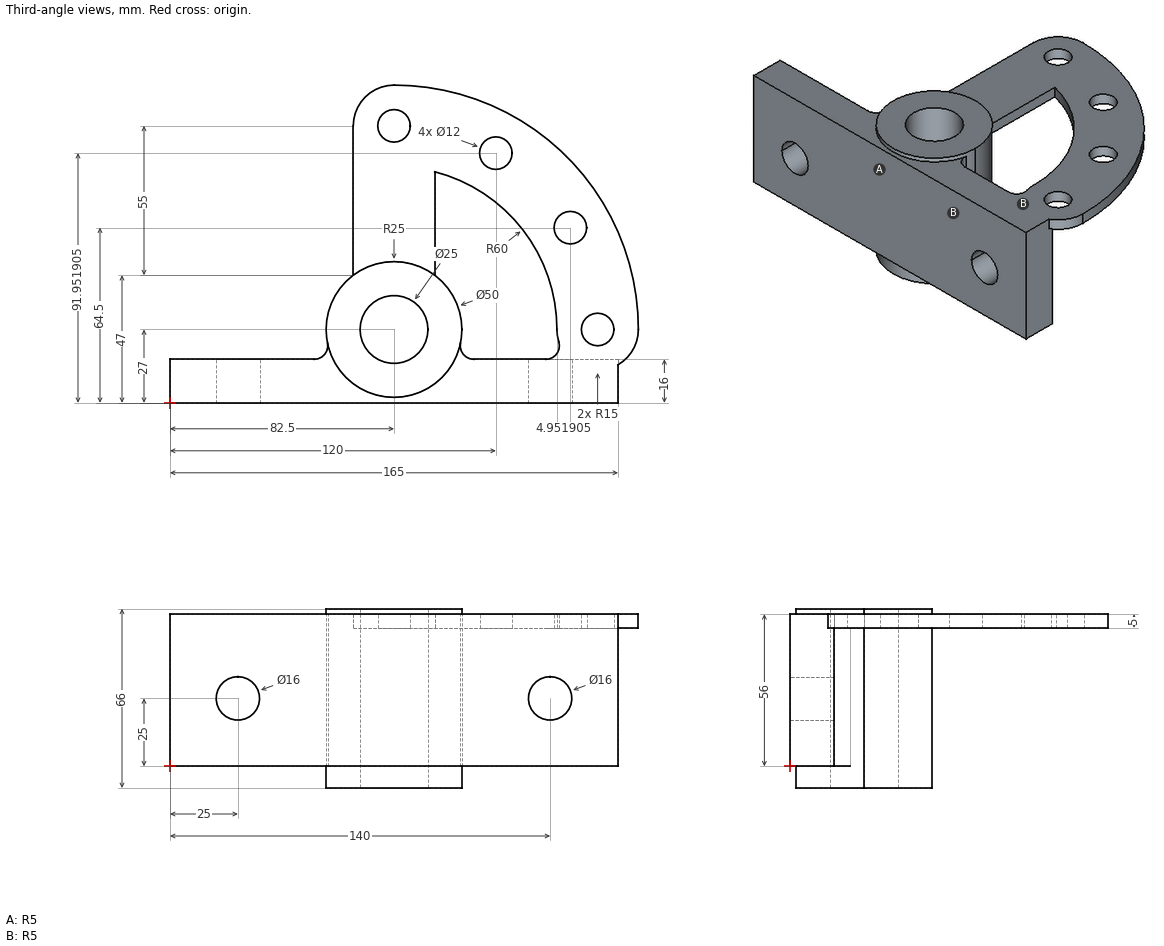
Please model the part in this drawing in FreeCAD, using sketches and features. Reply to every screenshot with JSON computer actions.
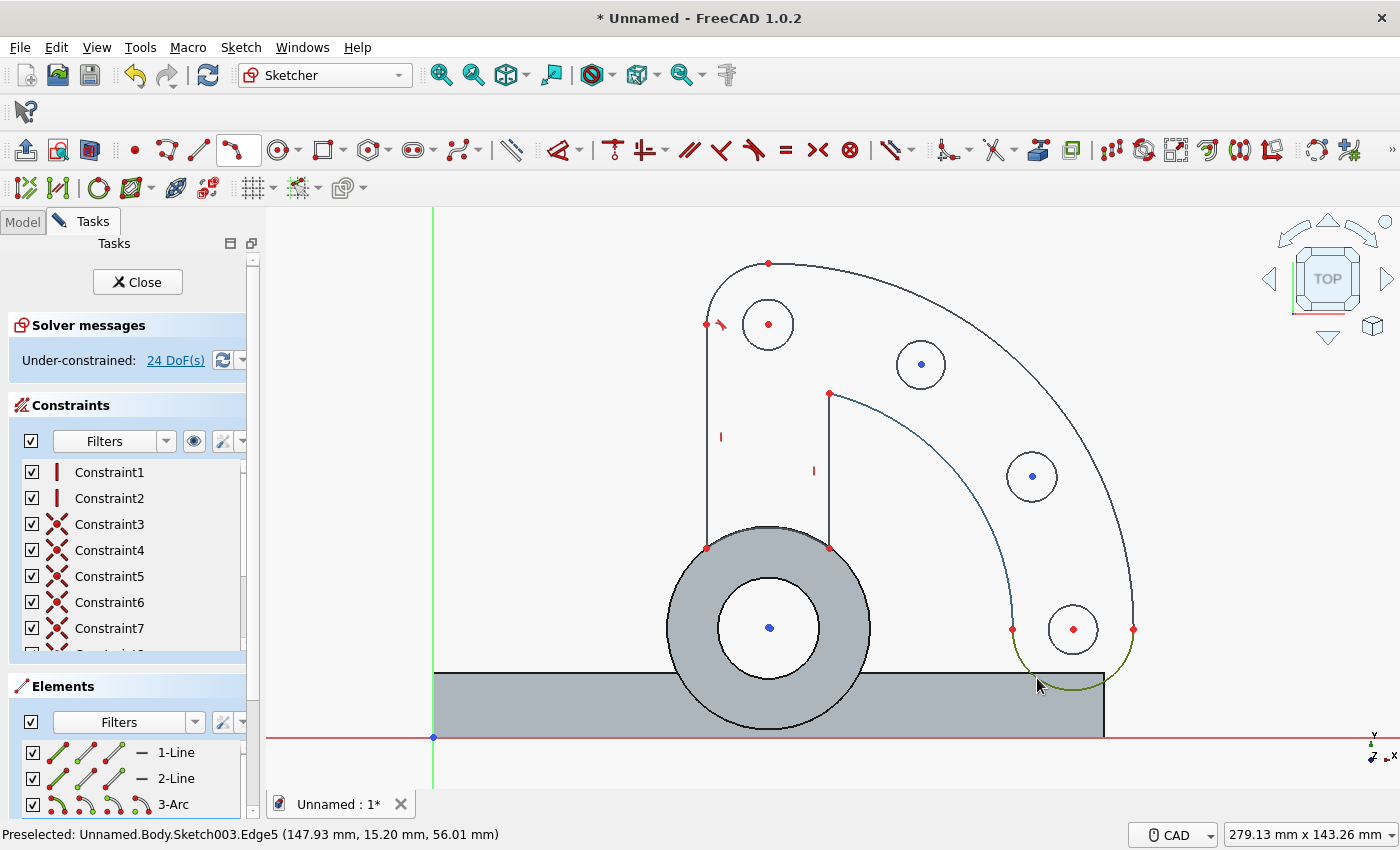
{"action": "left_click", "coordinate": [754, 150]}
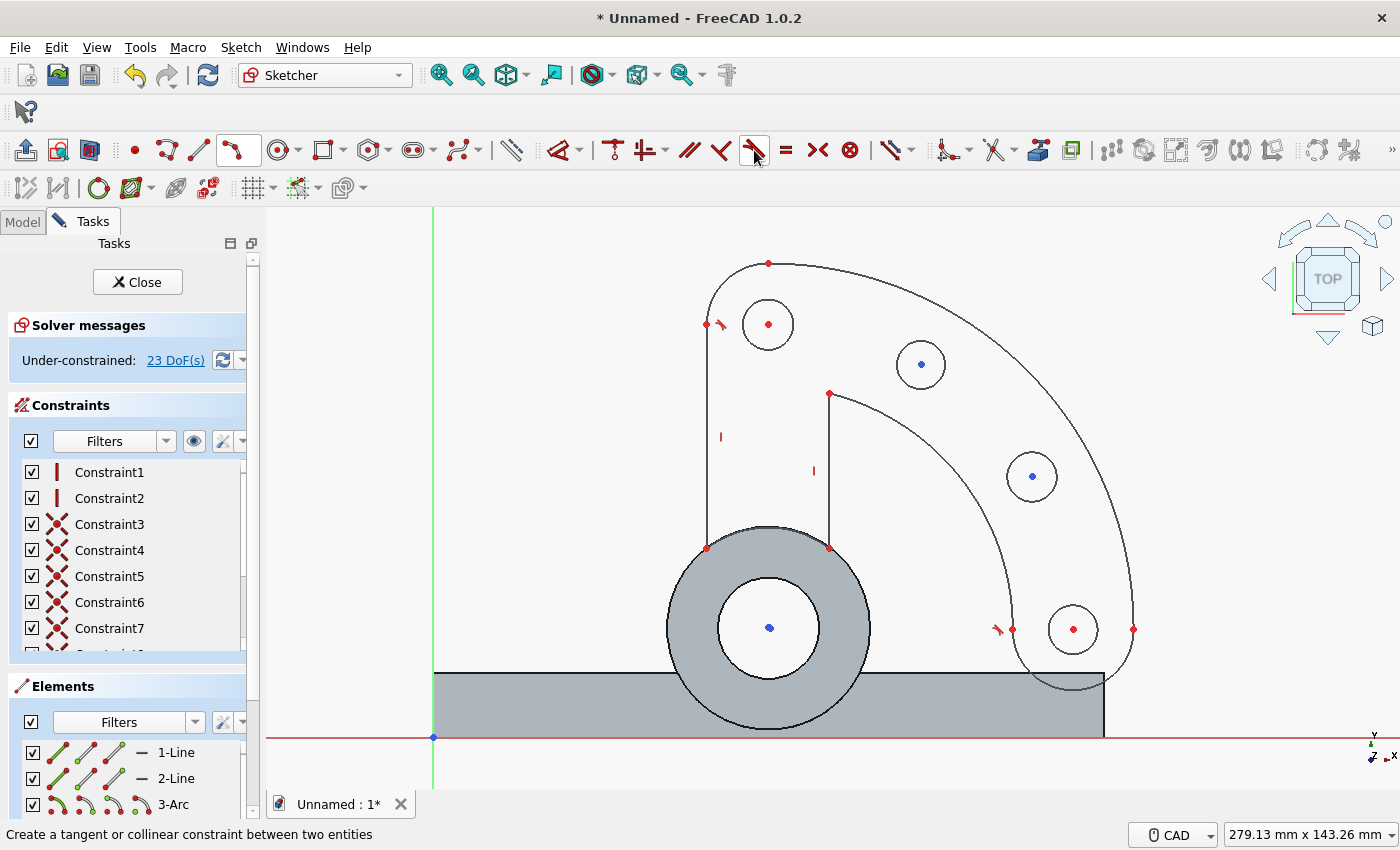
{"action": "left_click", "coordinate": [1038, 679]}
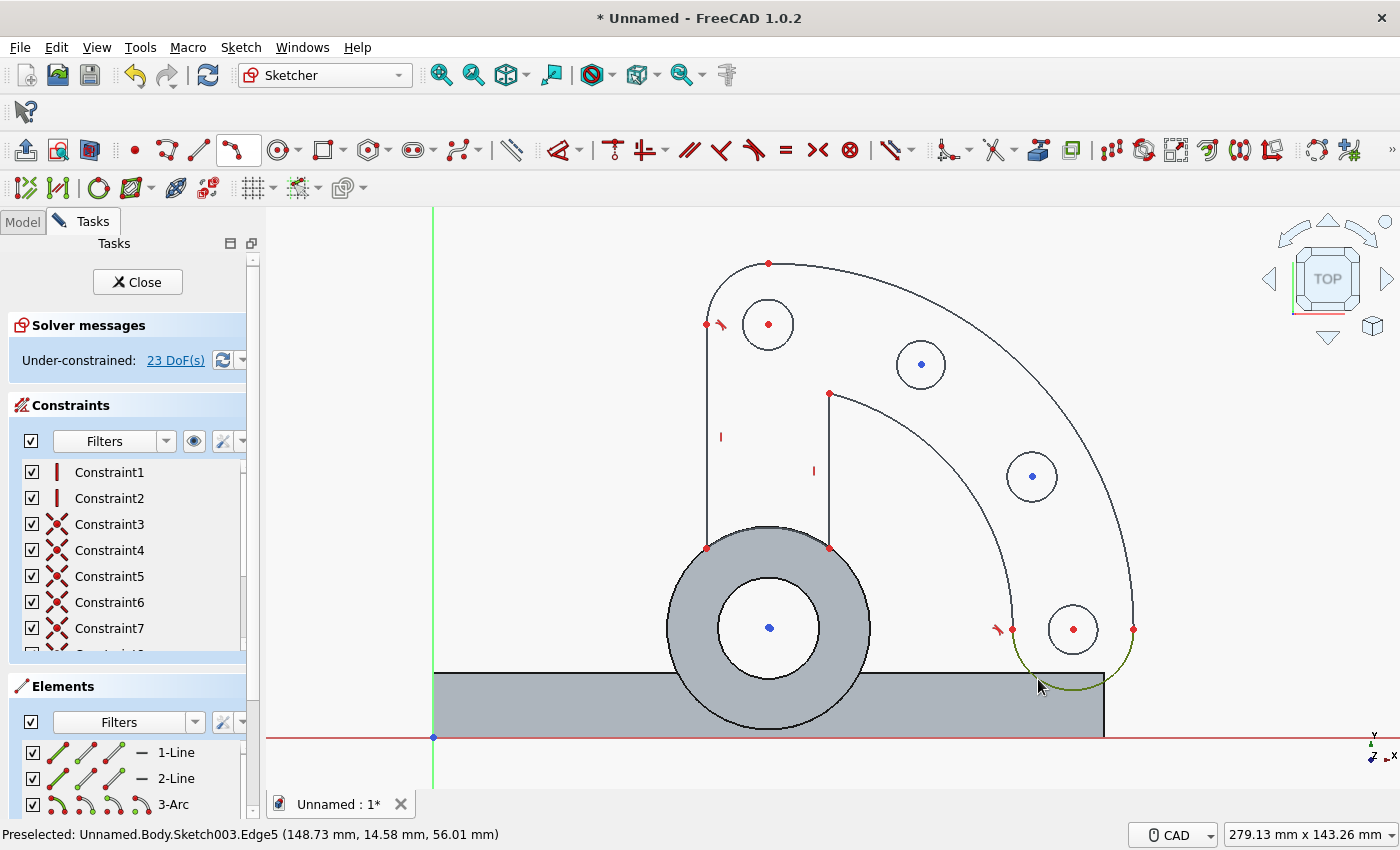
{"action": "left_click", "coordinate": [1094, 463]}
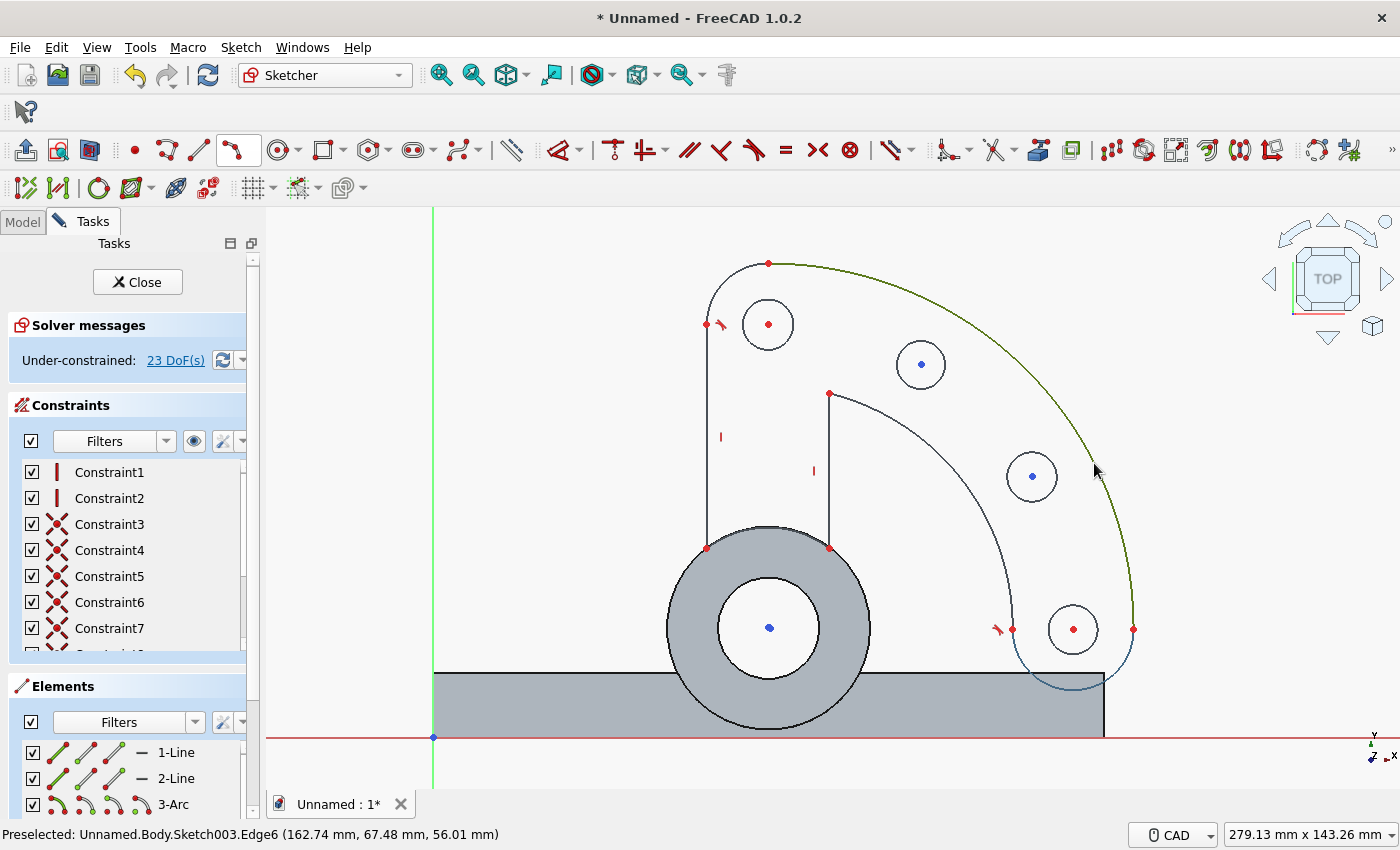
{"action": "left_click", "coordinate": [754, 150]}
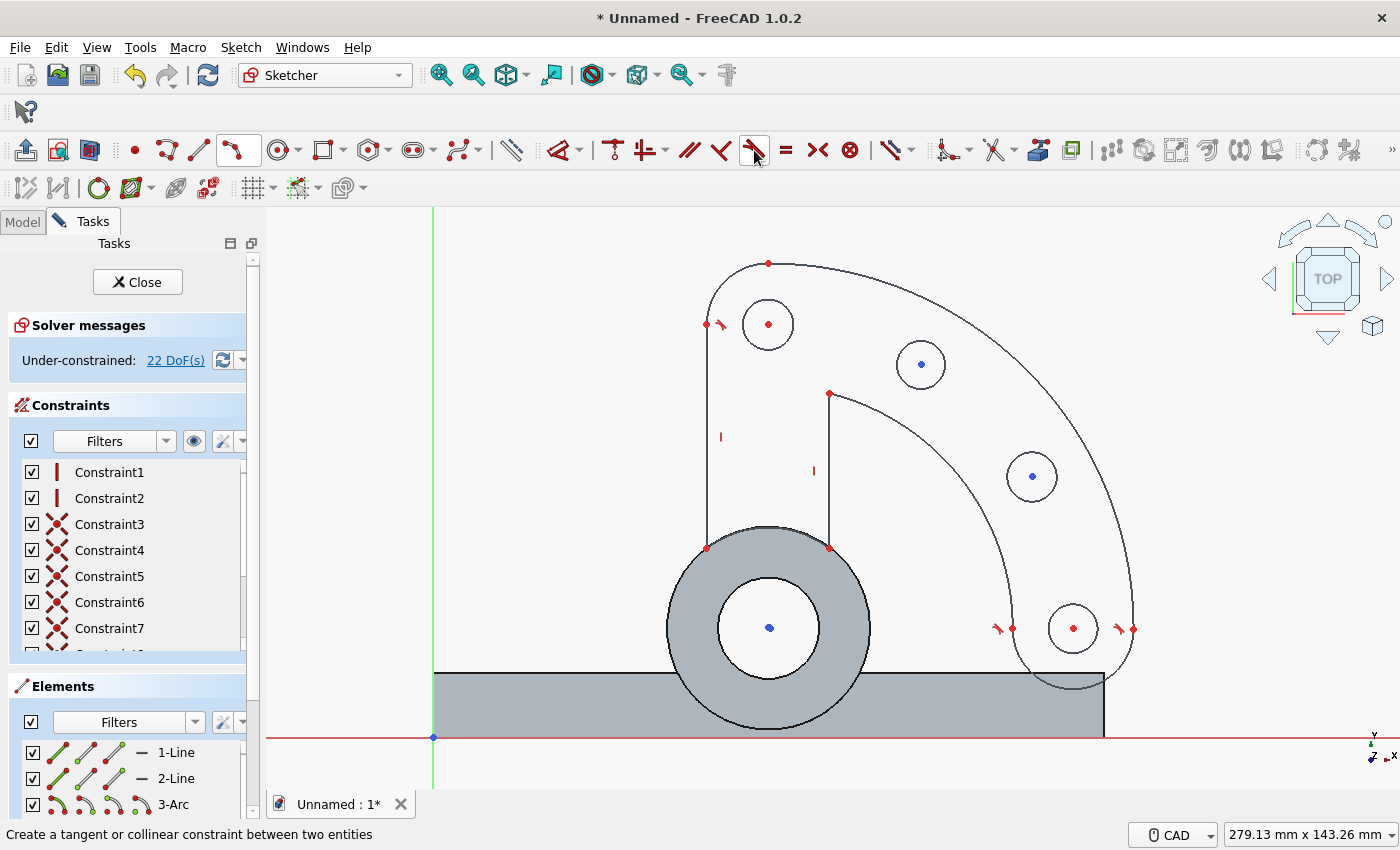
{"action": "left_click", "coordinate": [1094, 463]}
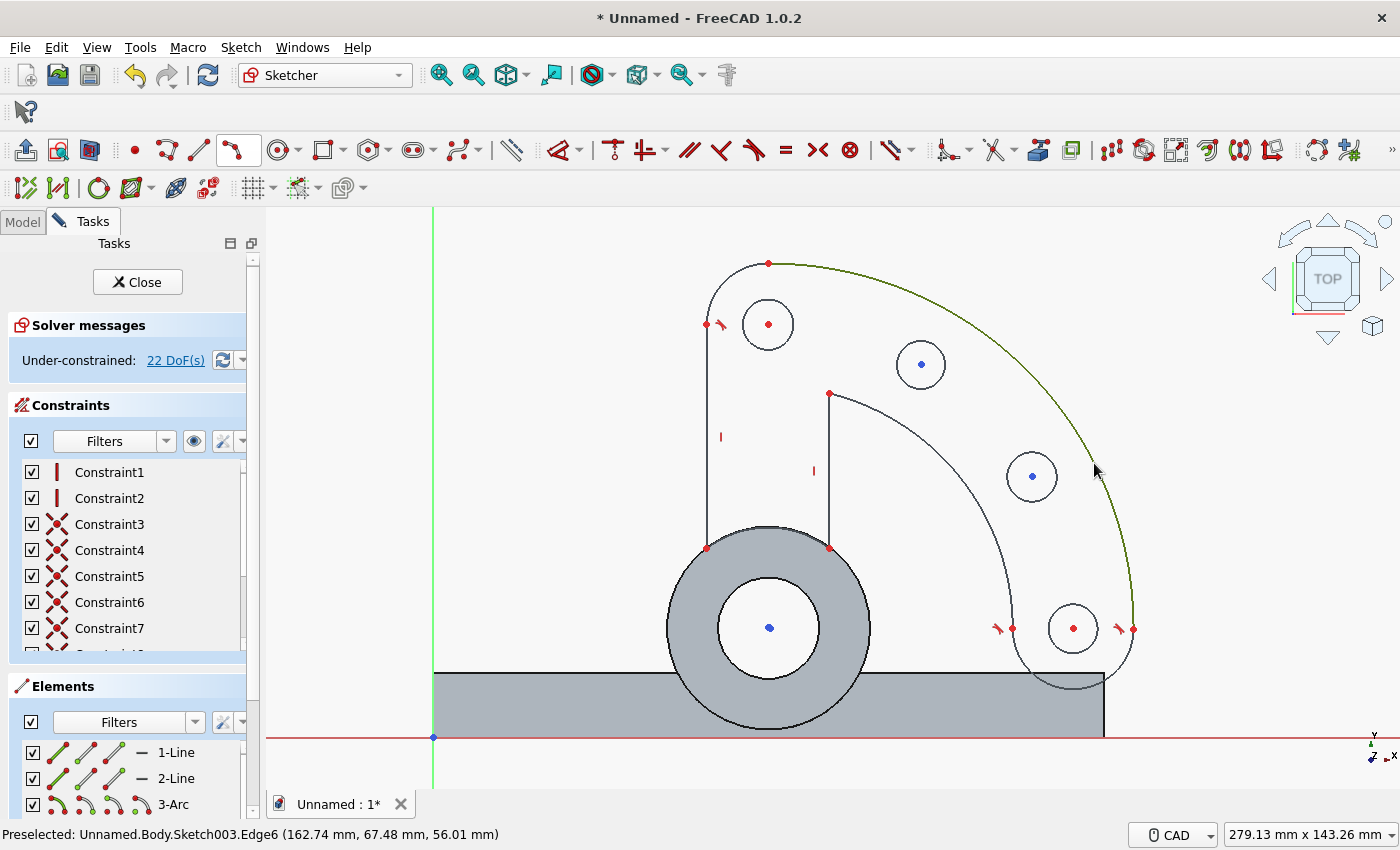
{"action": "left_click", "coordinate": [740, 270]}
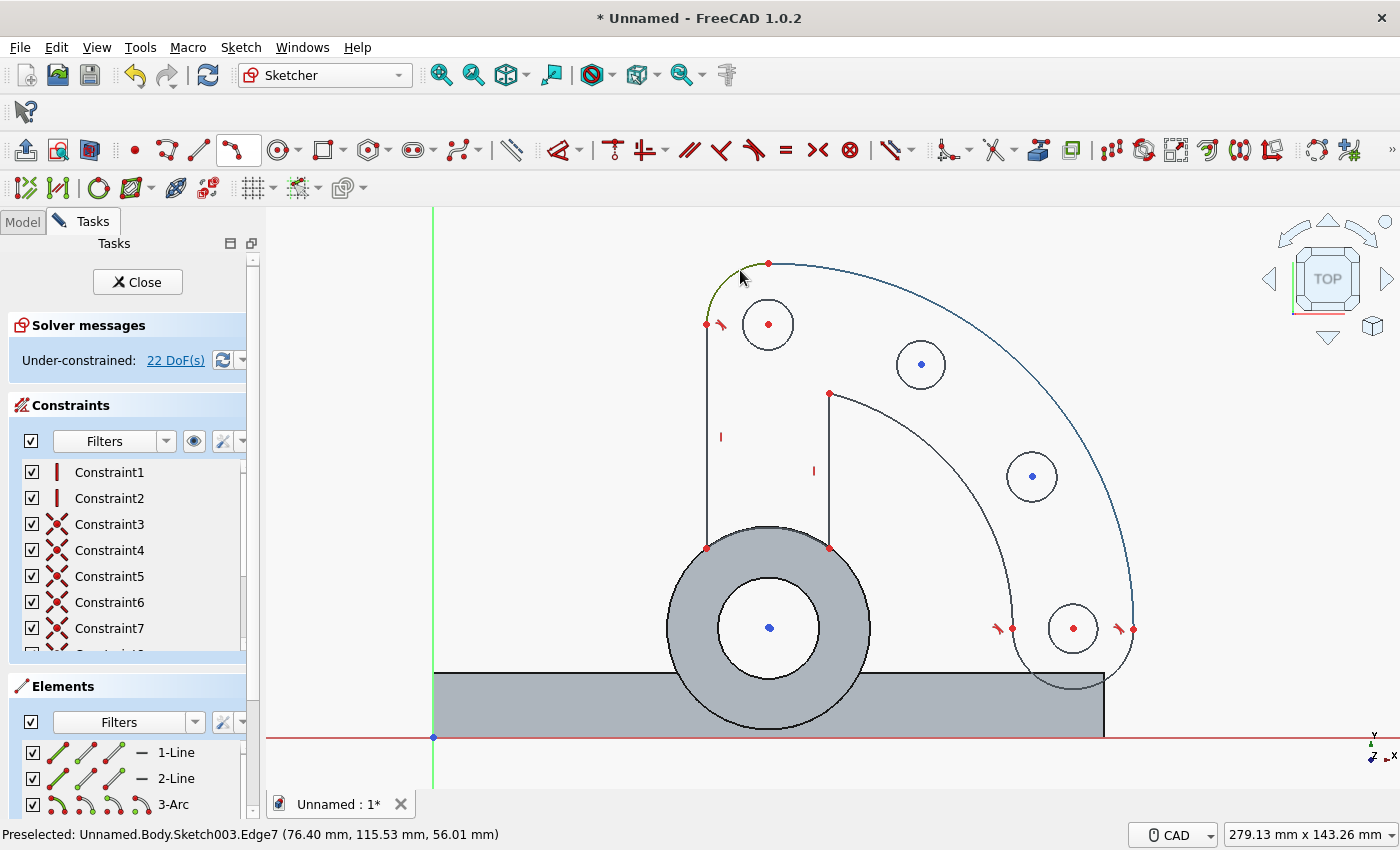
{"action": "key", "text": "t"}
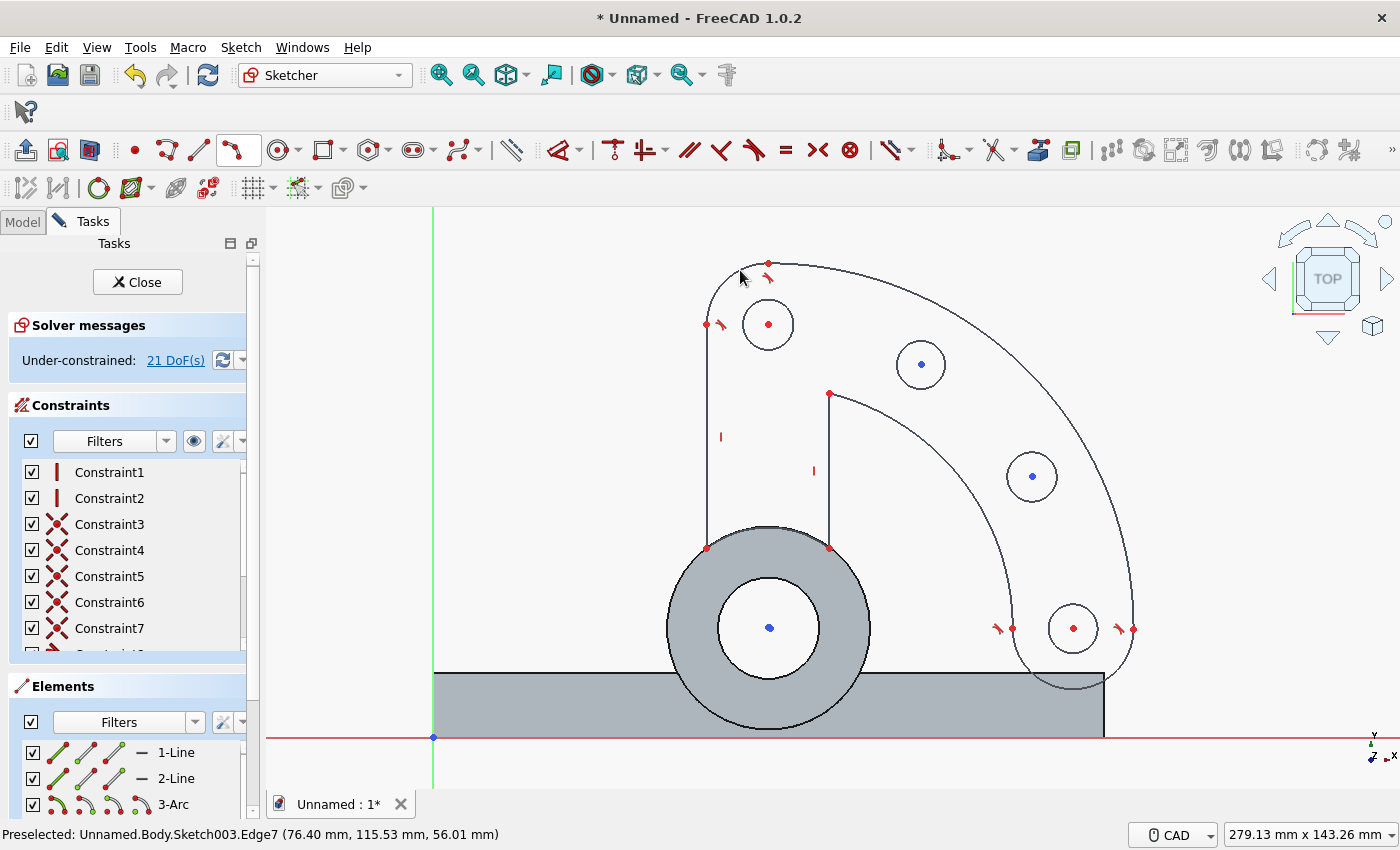
{"action": "left_click", "coordinate": [794, 531]}